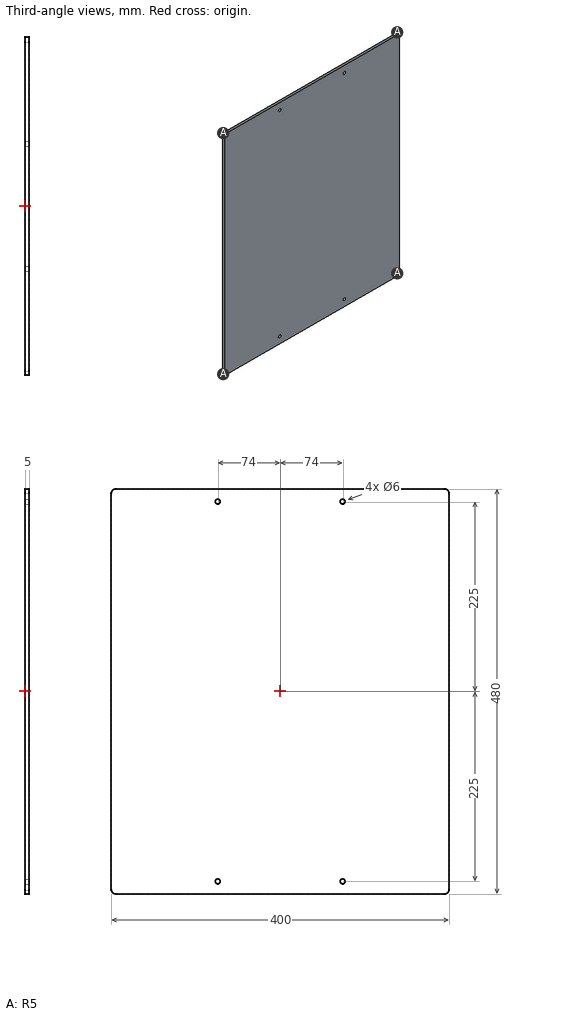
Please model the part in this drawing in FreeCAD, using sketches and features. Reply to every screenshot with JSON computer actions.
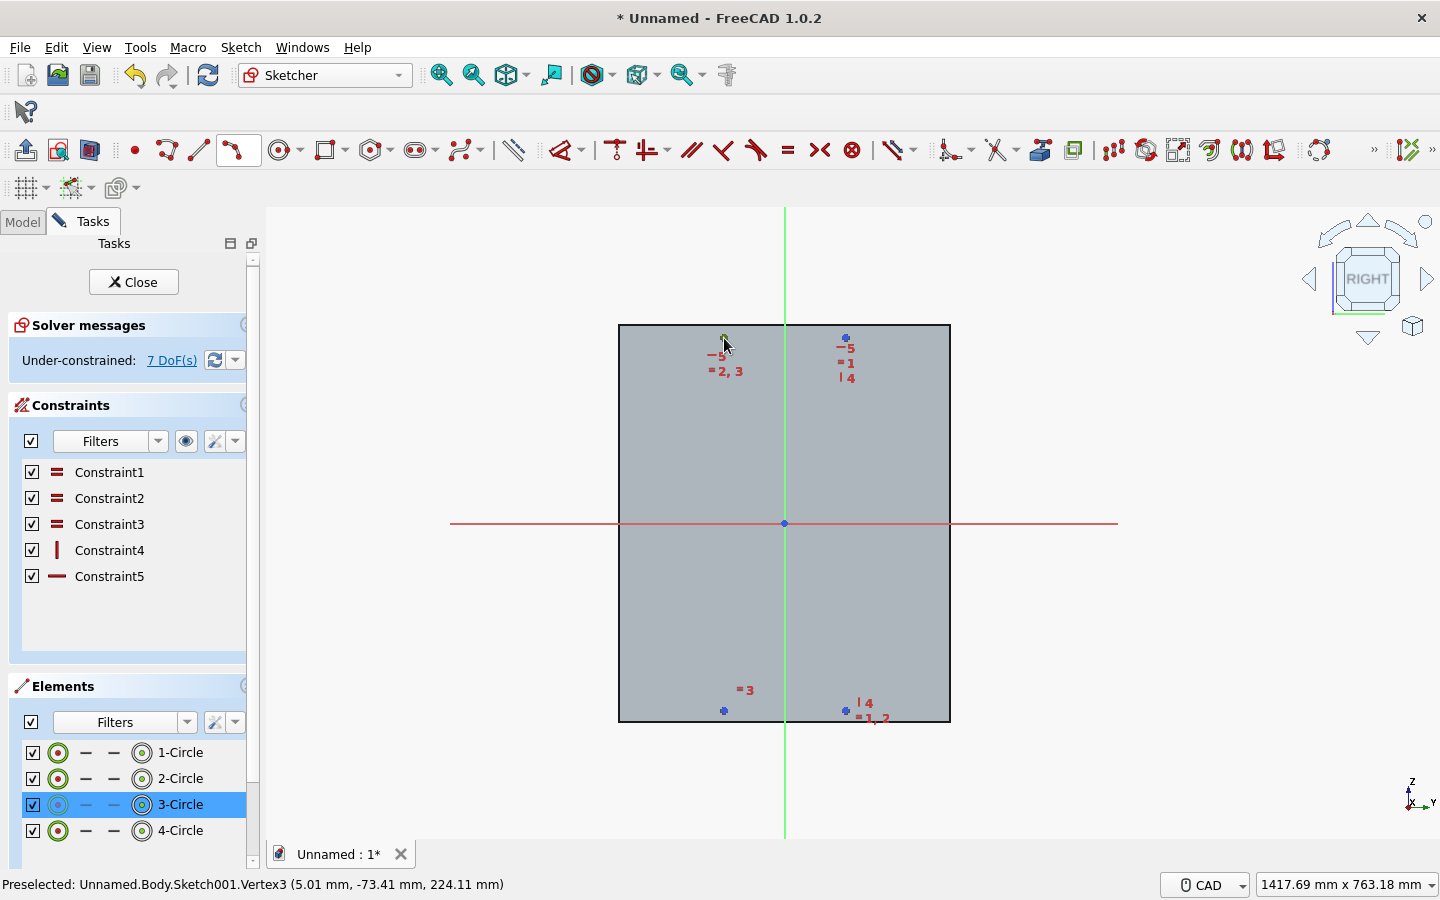
{"action": "left_click", "coordinate": [724, 711]}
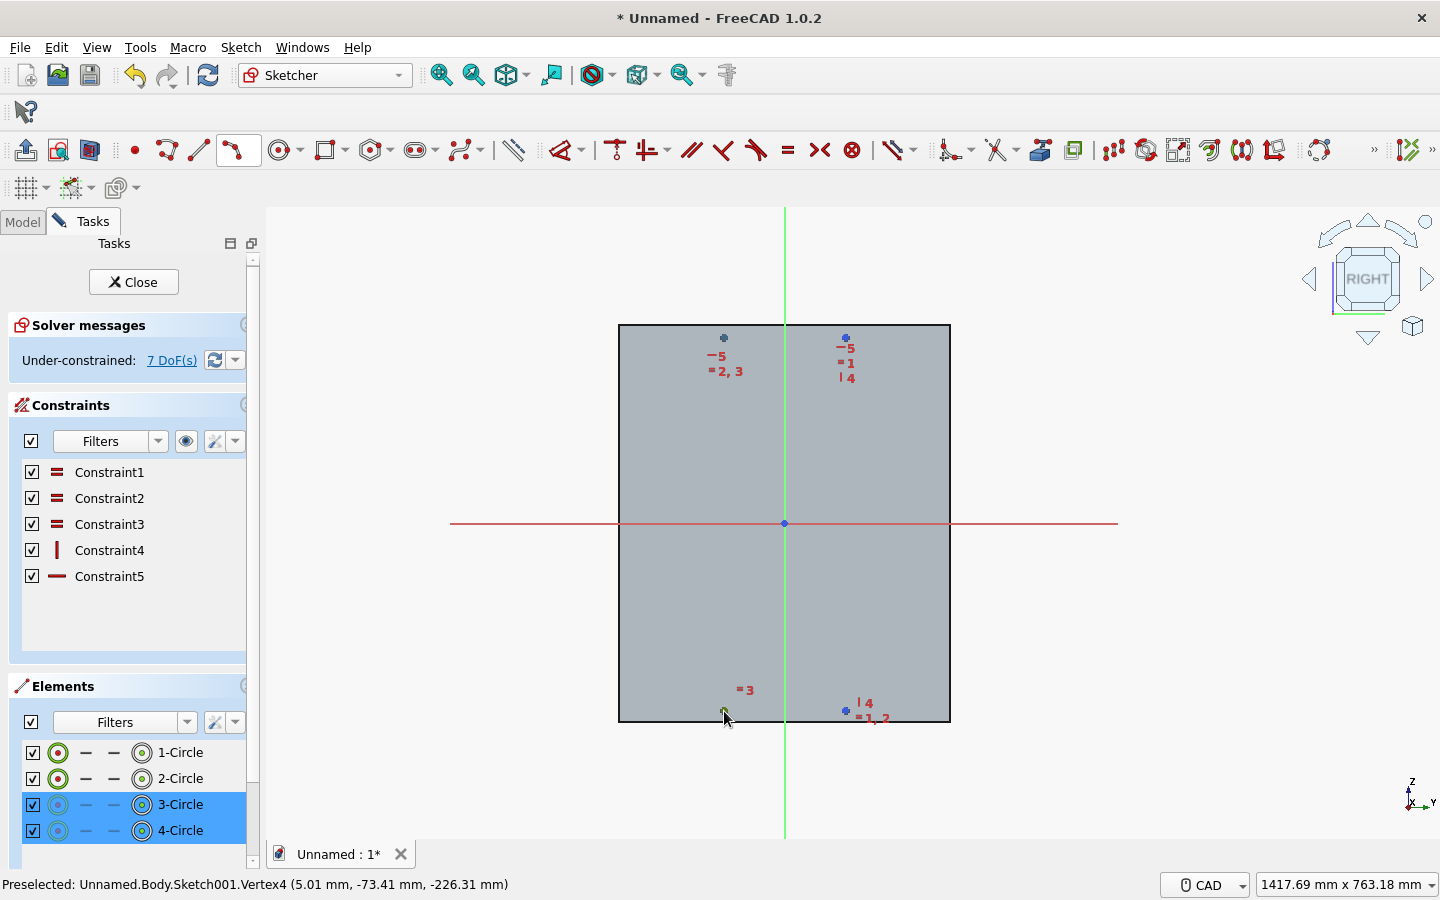
{"action": "key", "text": "v"}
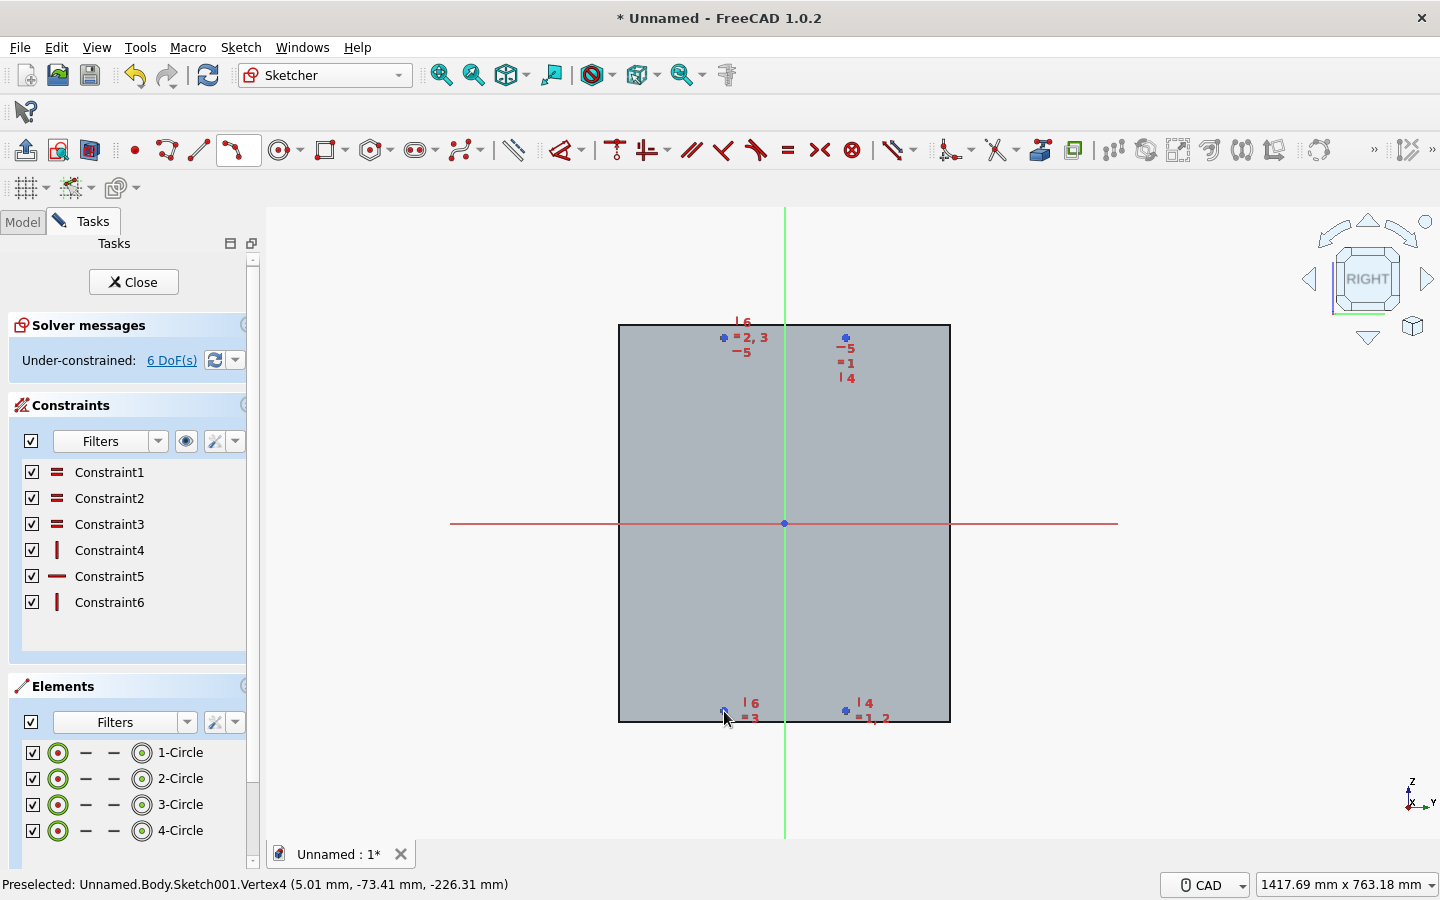
{"action": "left_click", "coordinate": [846, 711]}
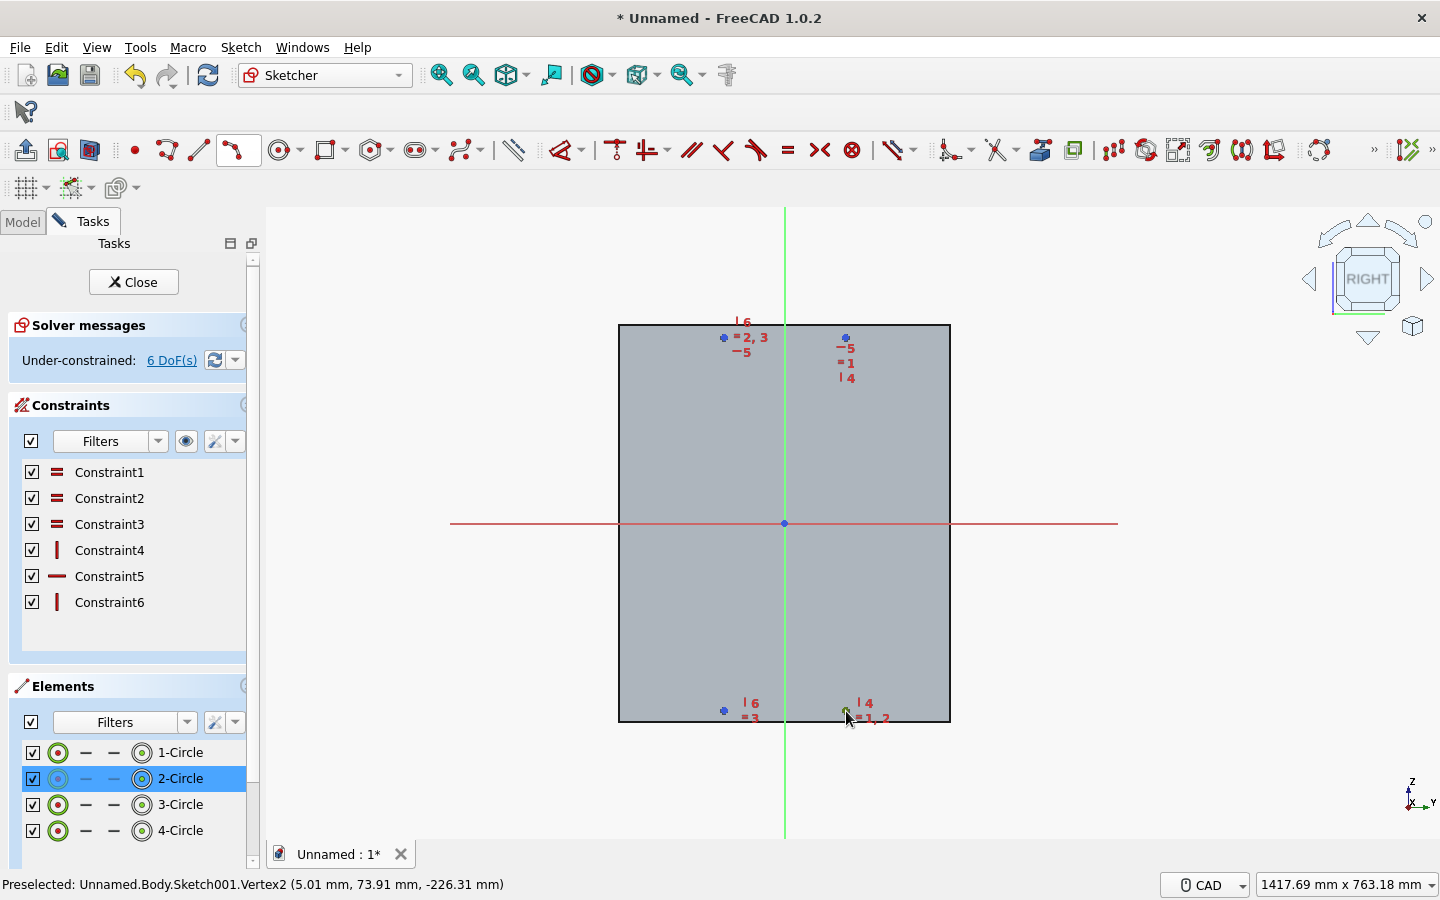
{"action": "left_click", "coordinate": [724, 711]}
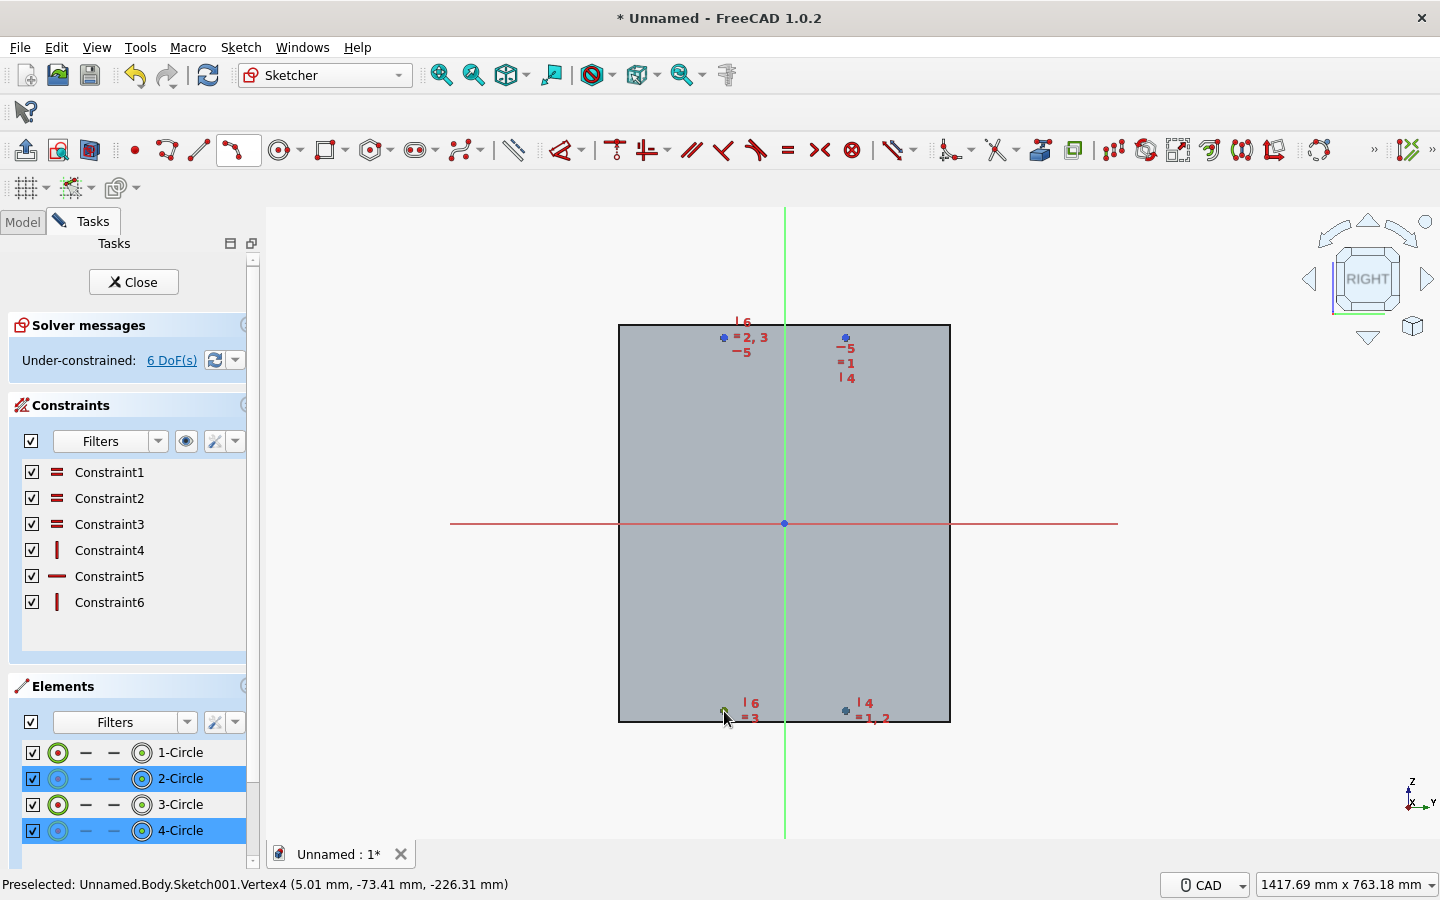
{"action": "key", "text": "h"}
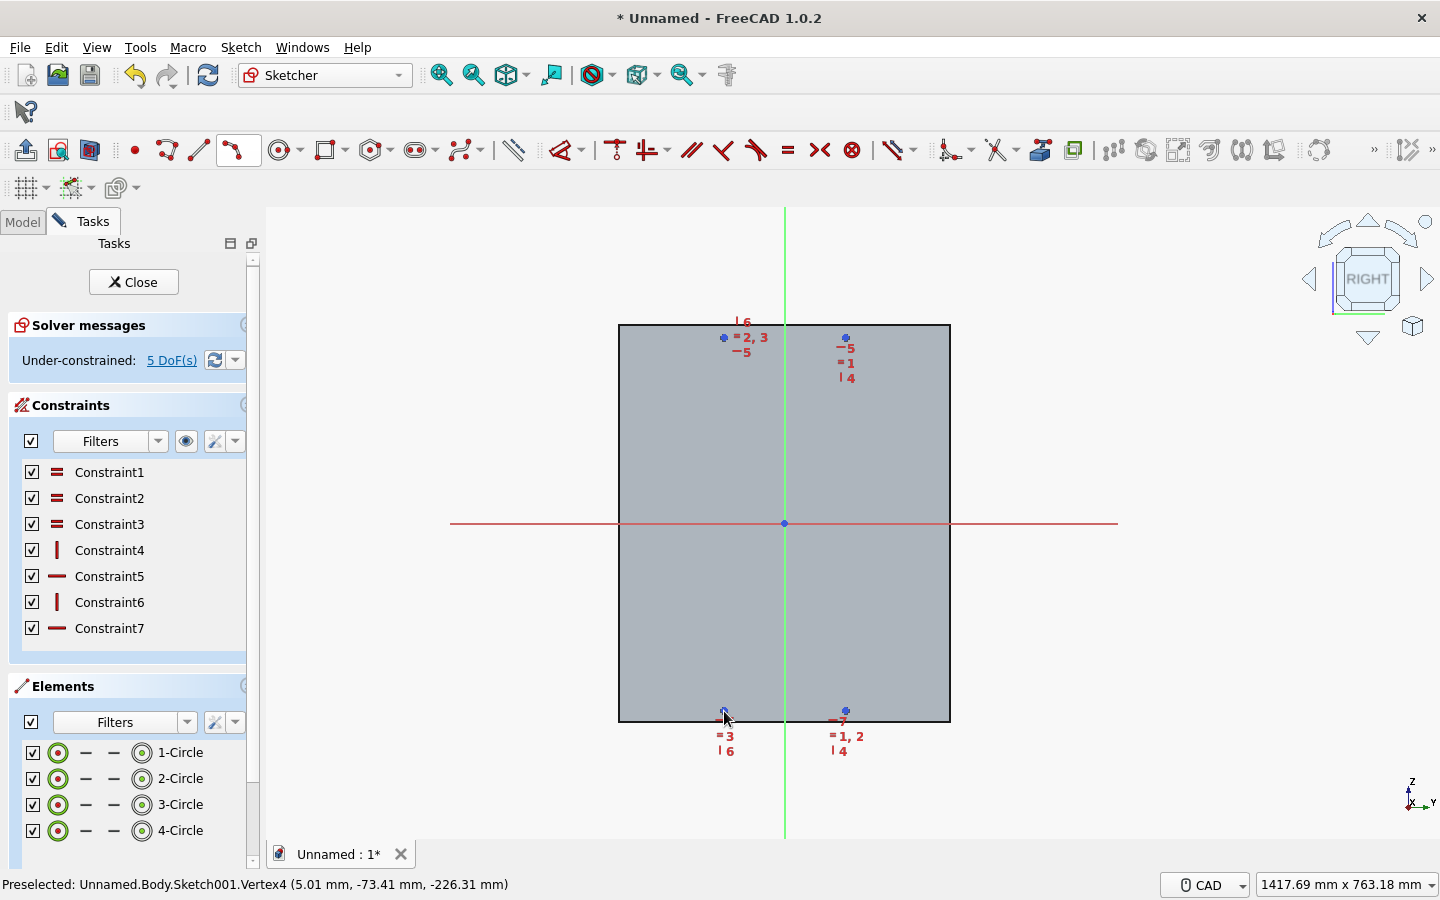
{"action": "left_click", "coordinate": [560, 150]}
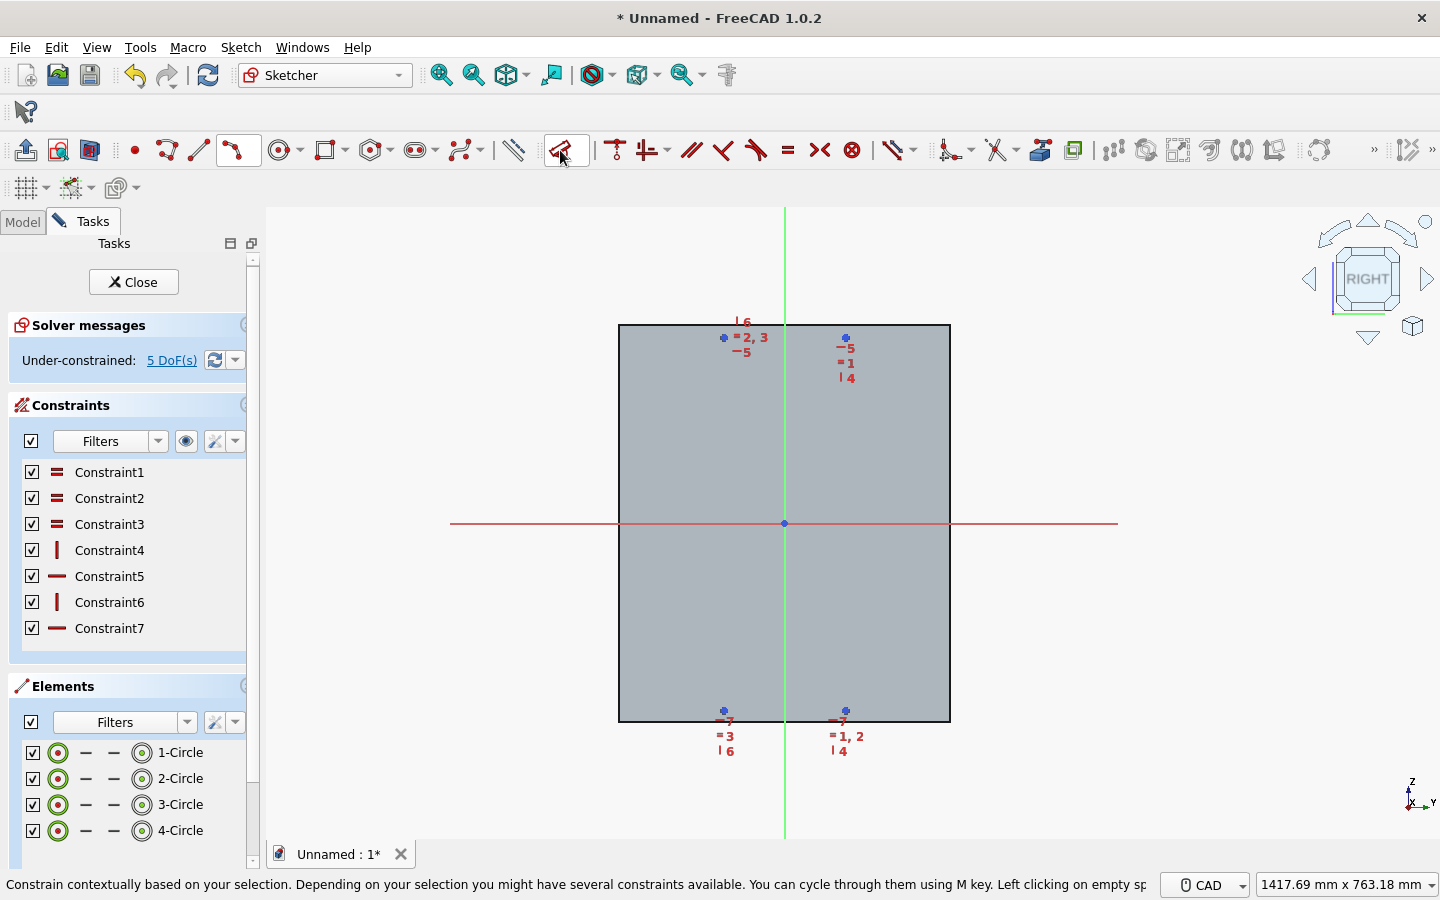
{"action": "scroll", "coordinate": [844, 336], "scroll_direction": "up", "scroll_amount": 11}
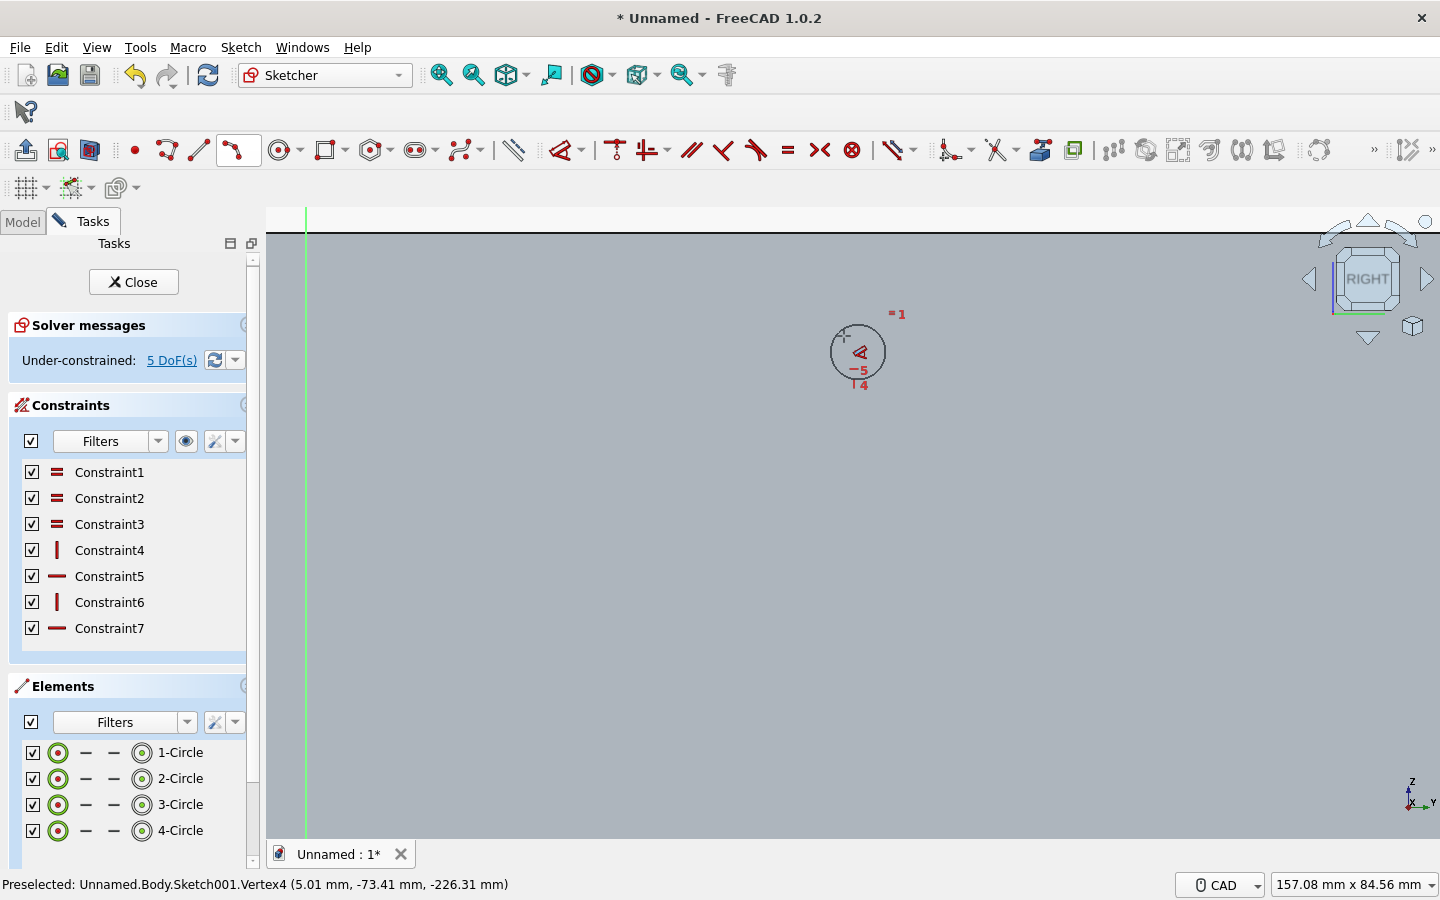
{"action": "left_click", "coordinate": [839, 333]}
{"action": "left_click", "coordinate": [816, 310]}